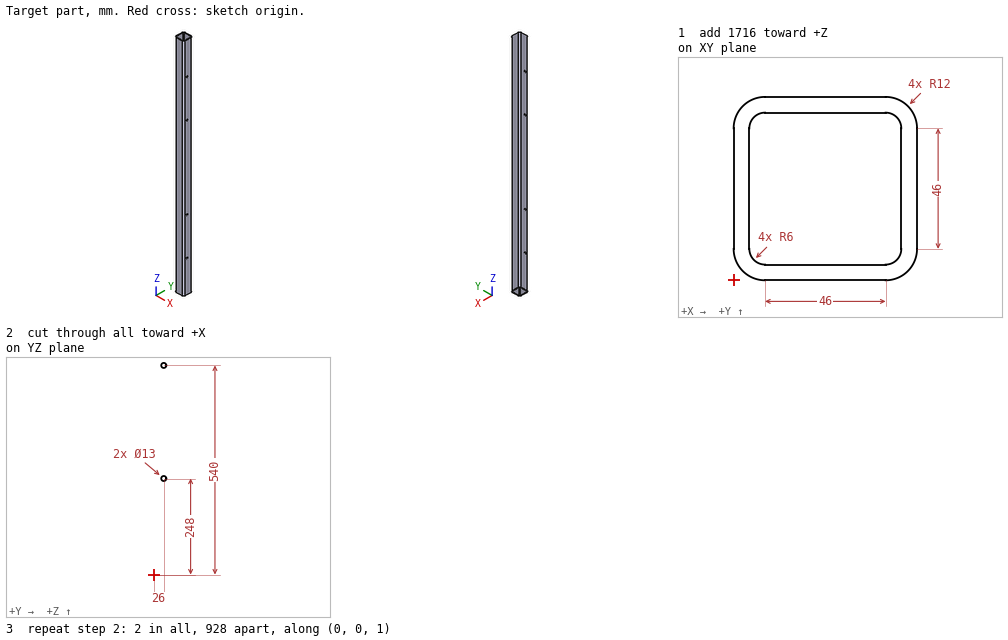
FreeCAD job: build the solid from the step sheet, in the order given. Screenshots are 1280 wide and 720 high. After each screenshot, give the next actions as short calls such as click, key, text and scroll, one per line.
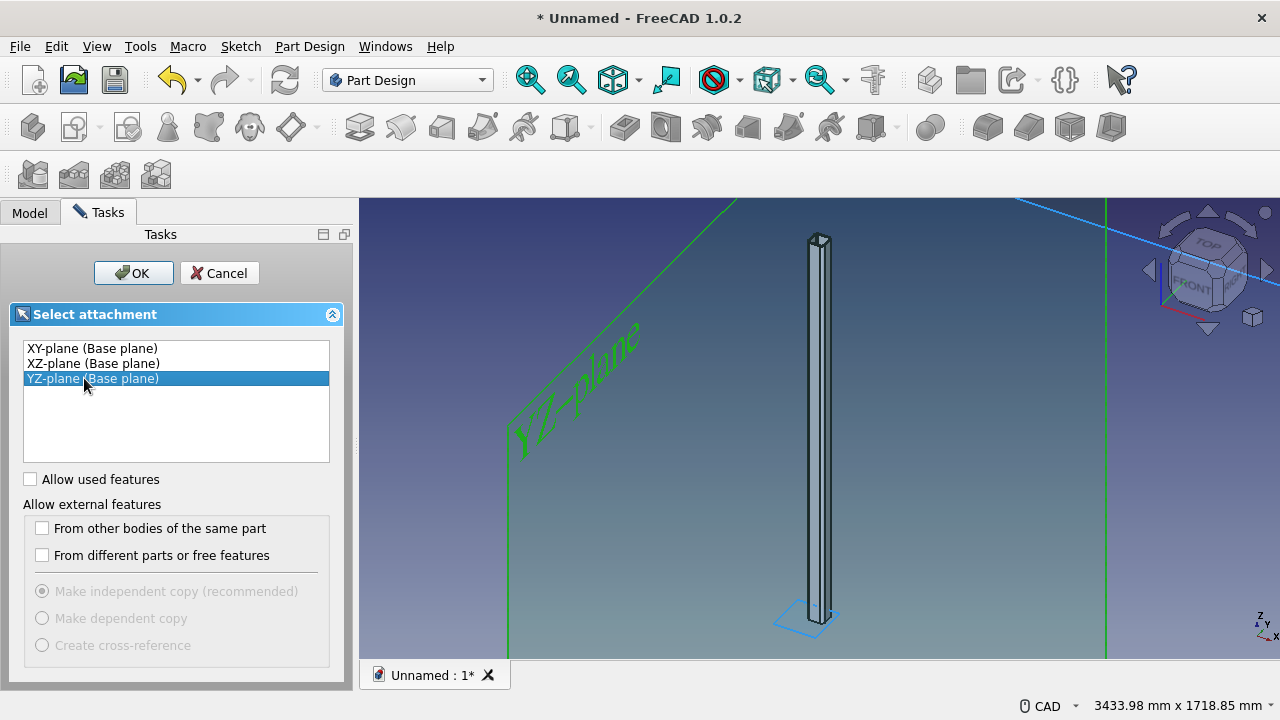
click(134, 273)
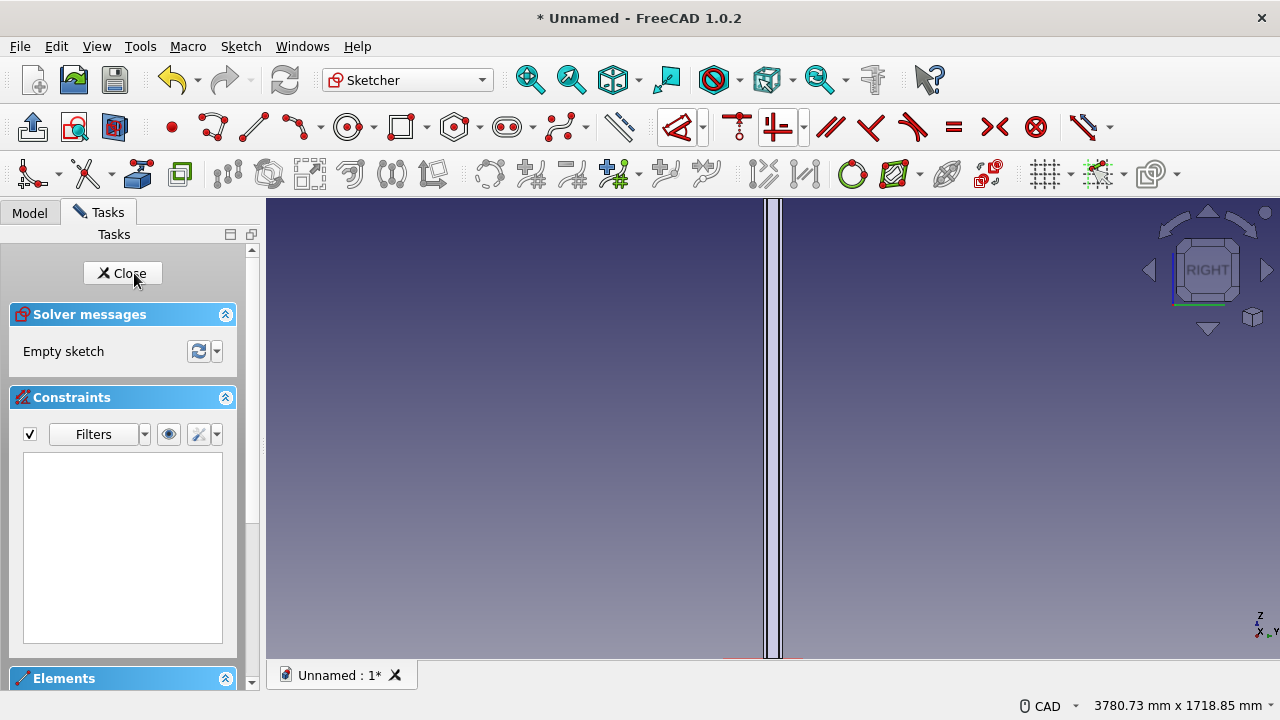
click(115, 128)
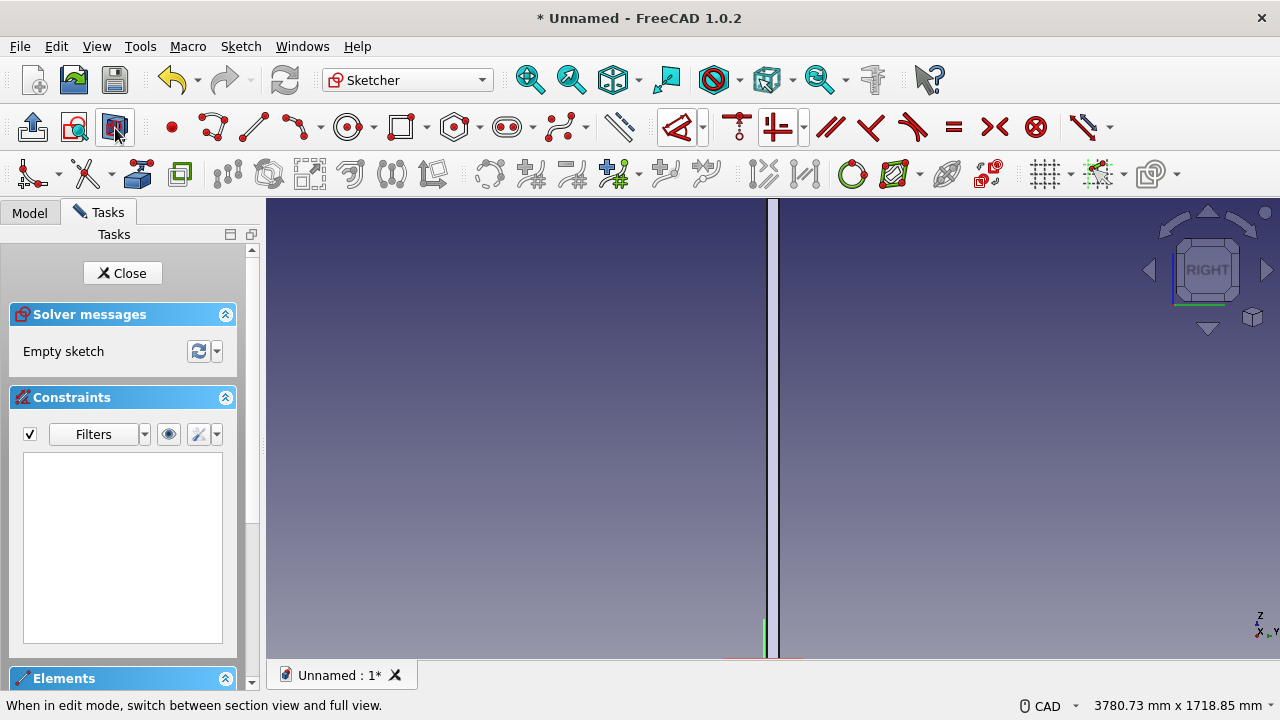
scroll(704, 428, down, 5)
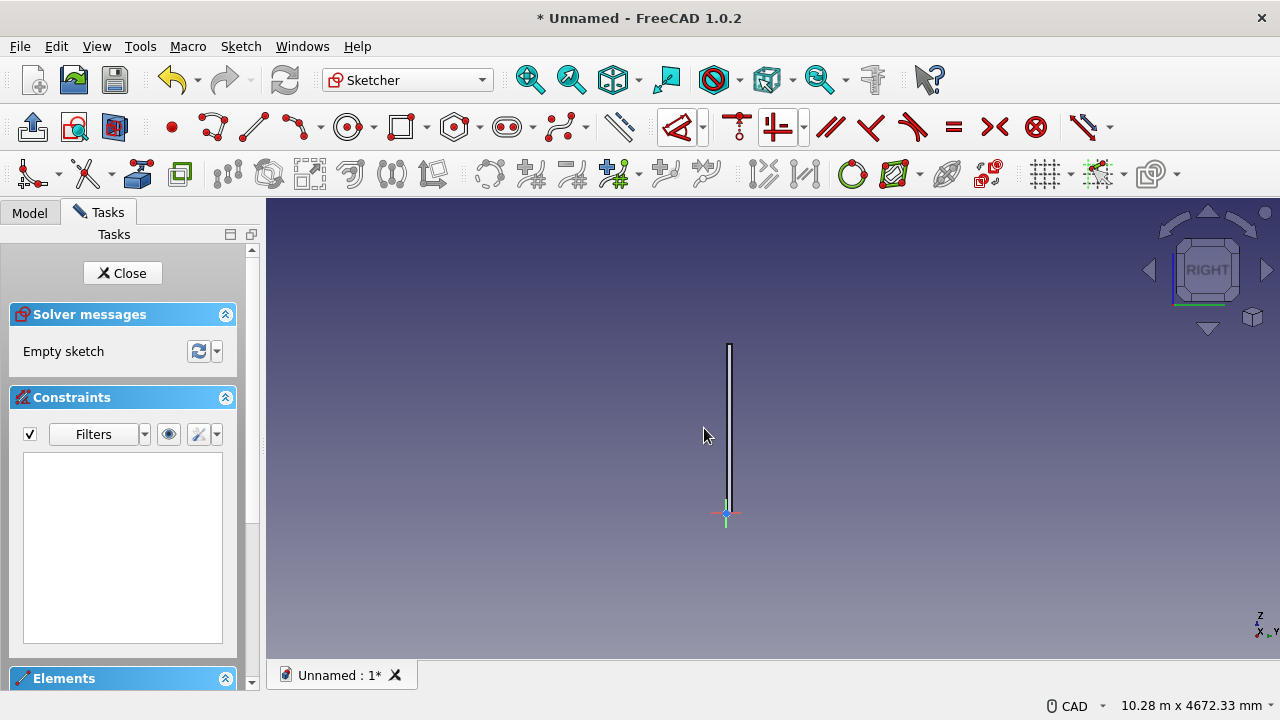
scroll(734, 501, up, 8)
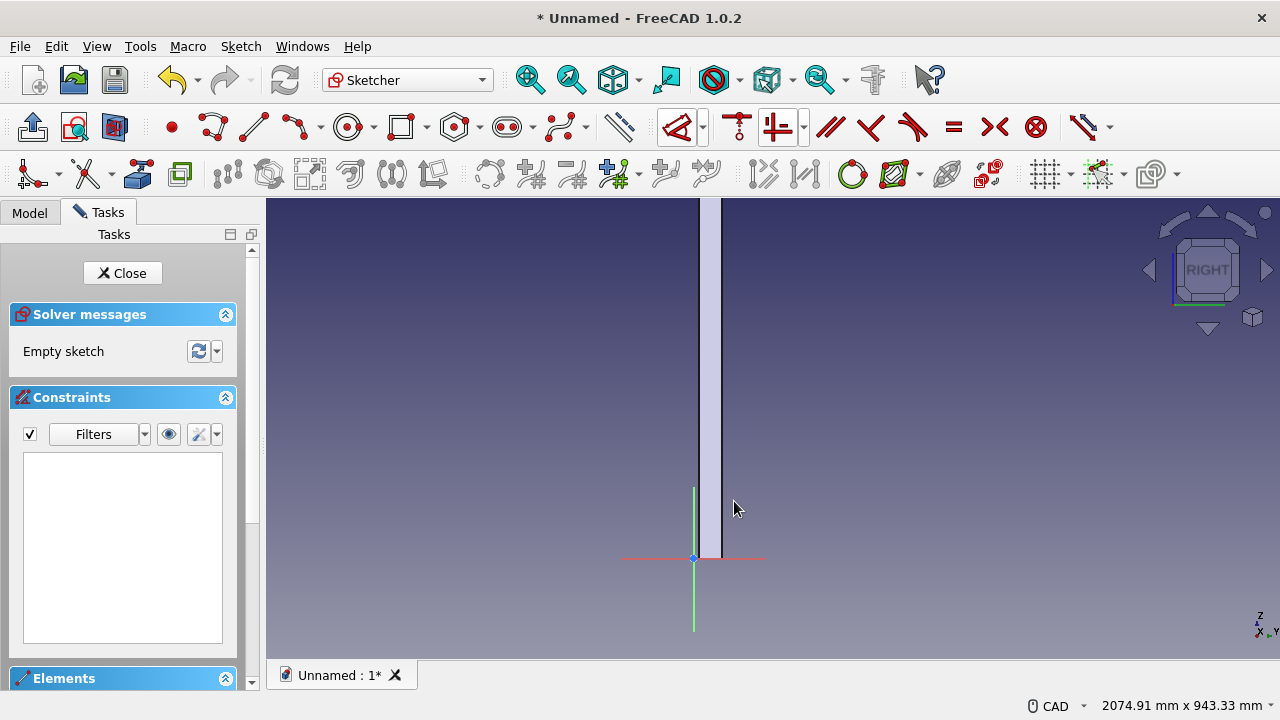
click(348, 128)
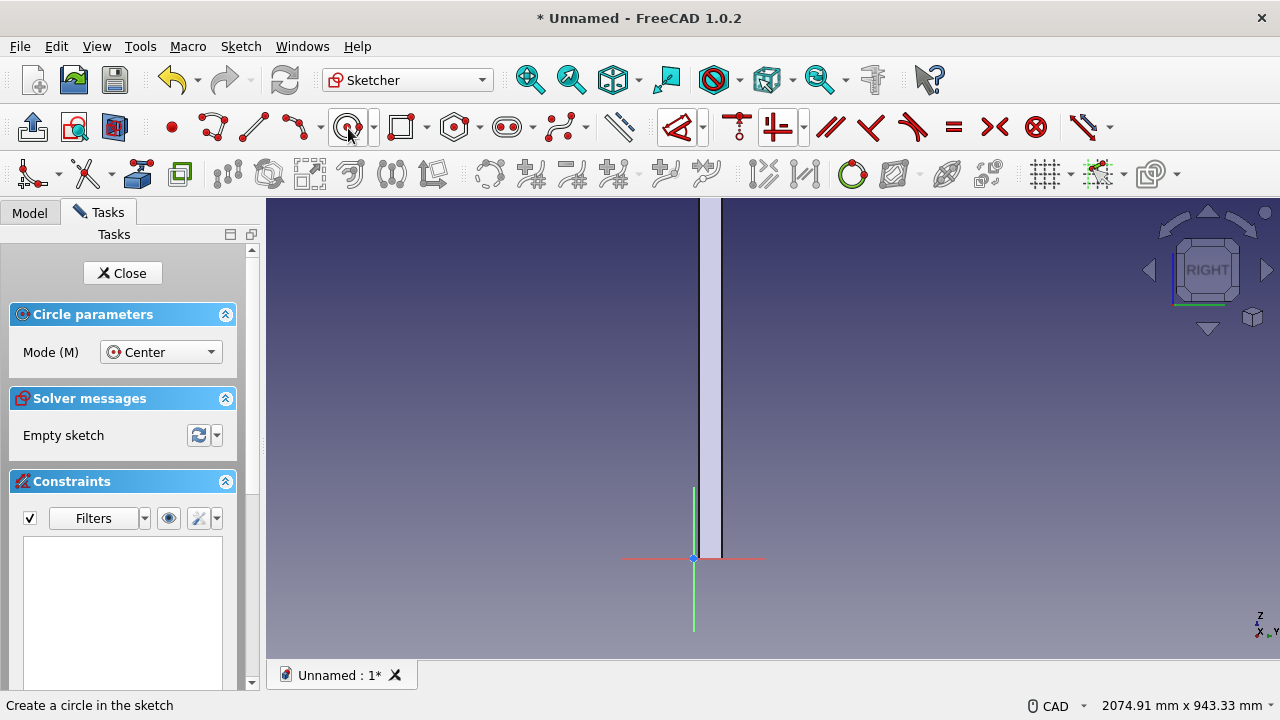
scroll(706, 437, up, 10)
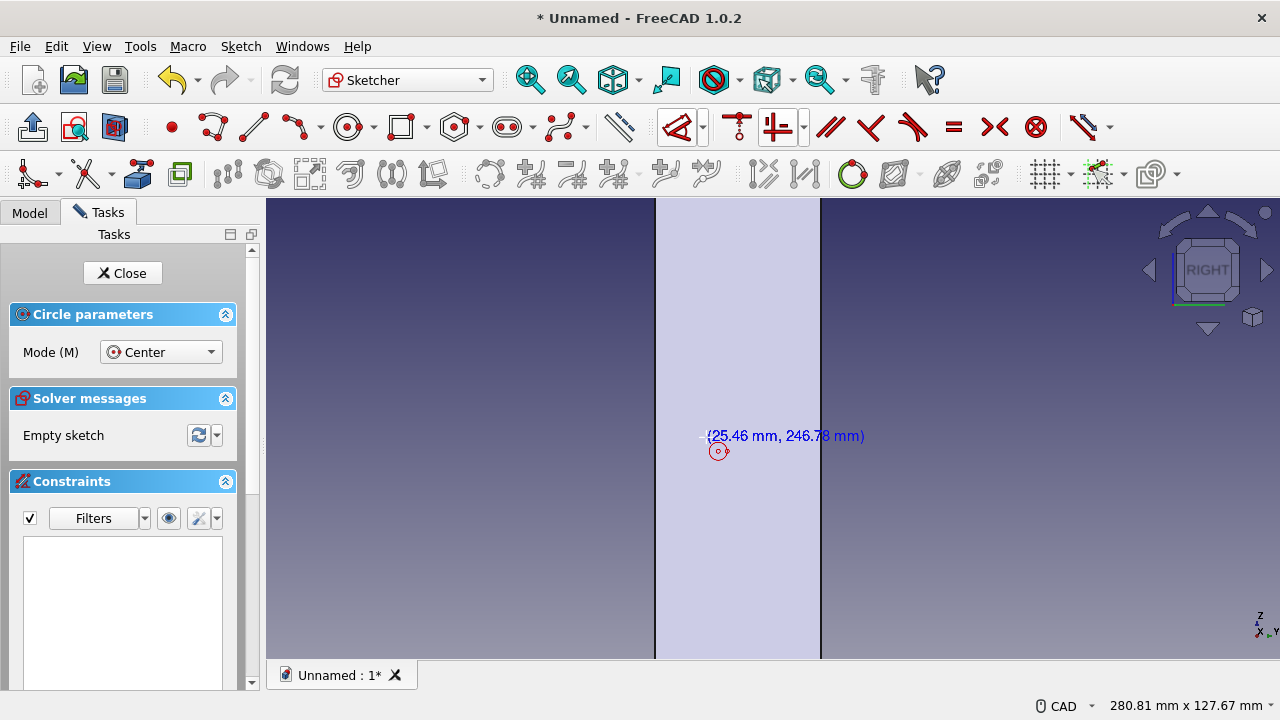
scroll(710, 441, down, 10)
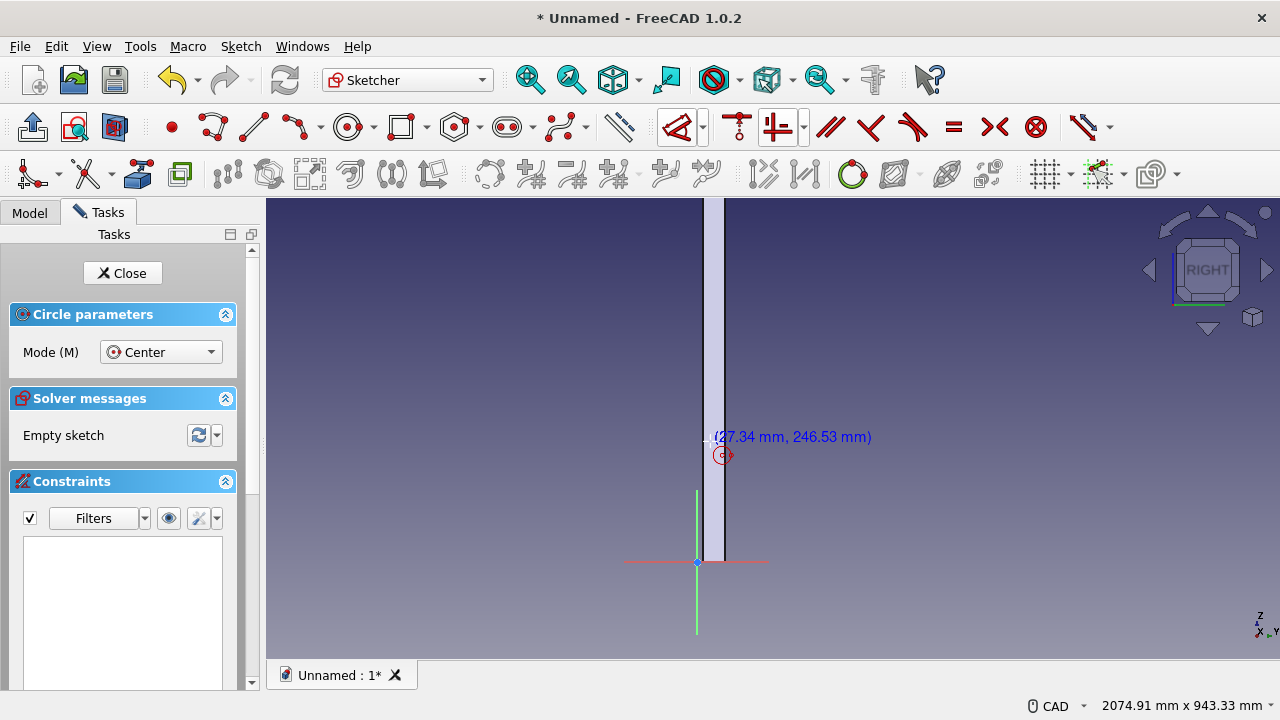
scroll(710, 441, up, 2)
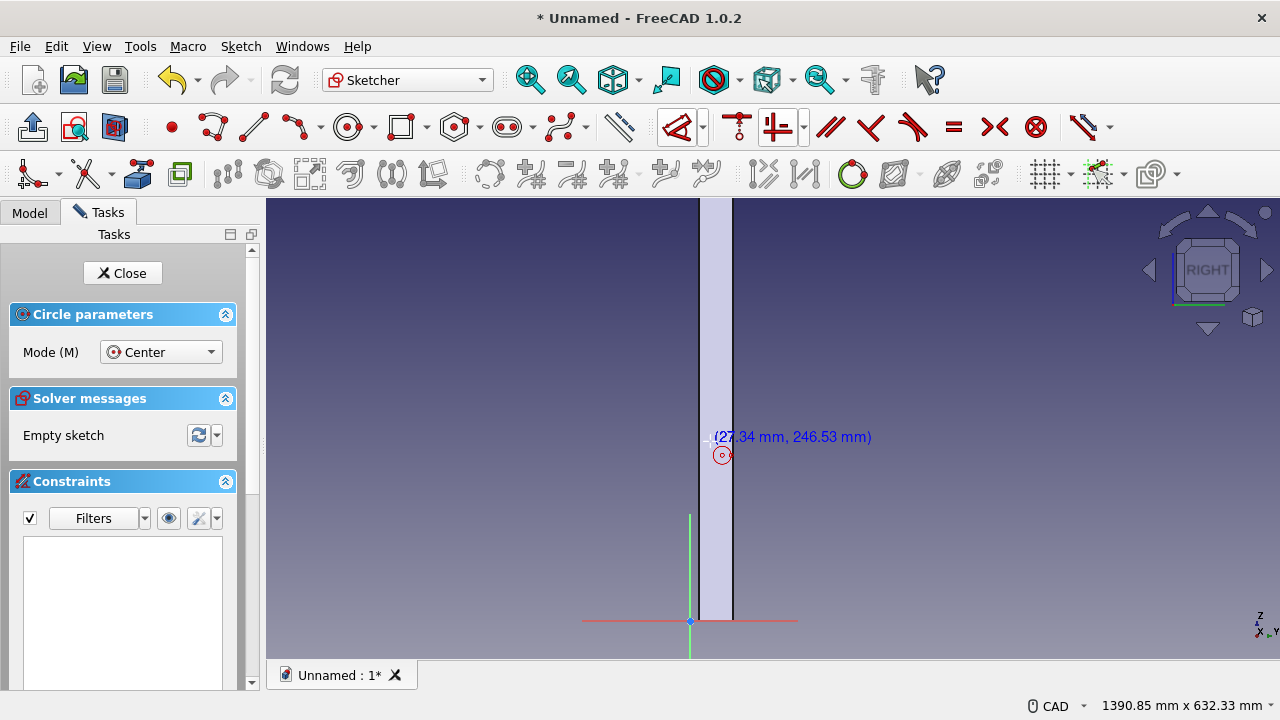
click(709, 441)
move(713, 437)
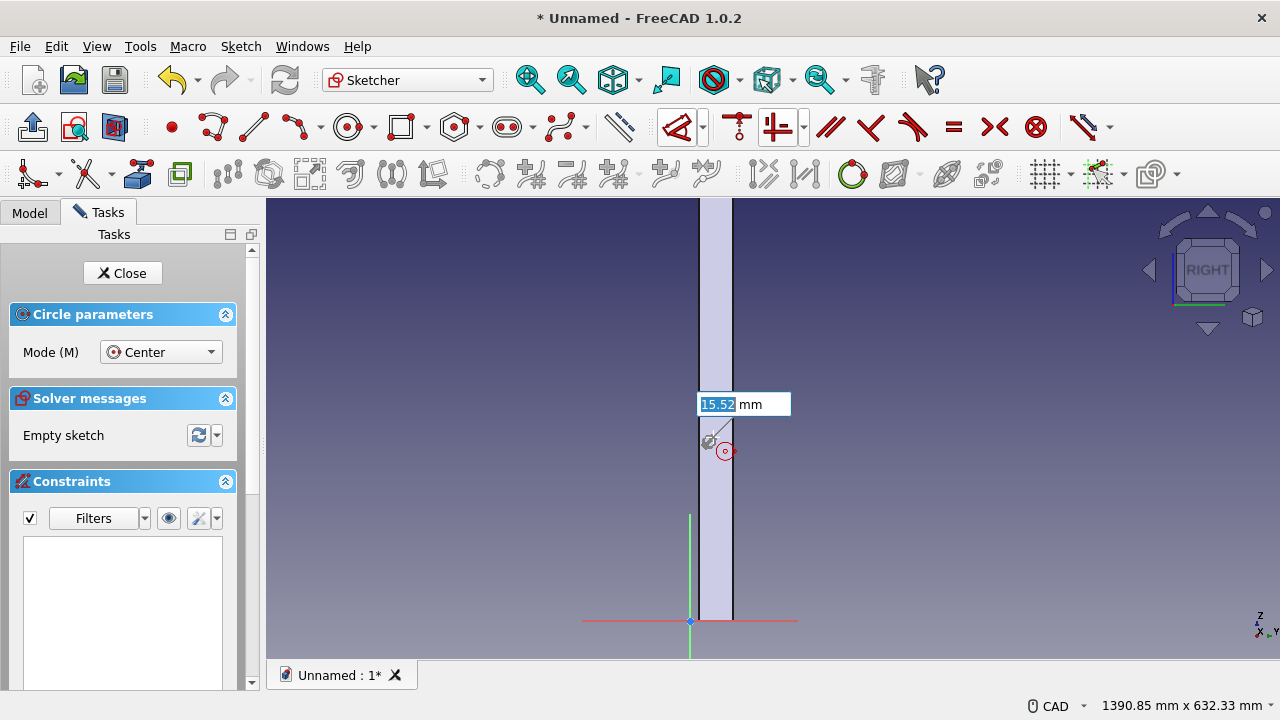
text(13)
key(Return)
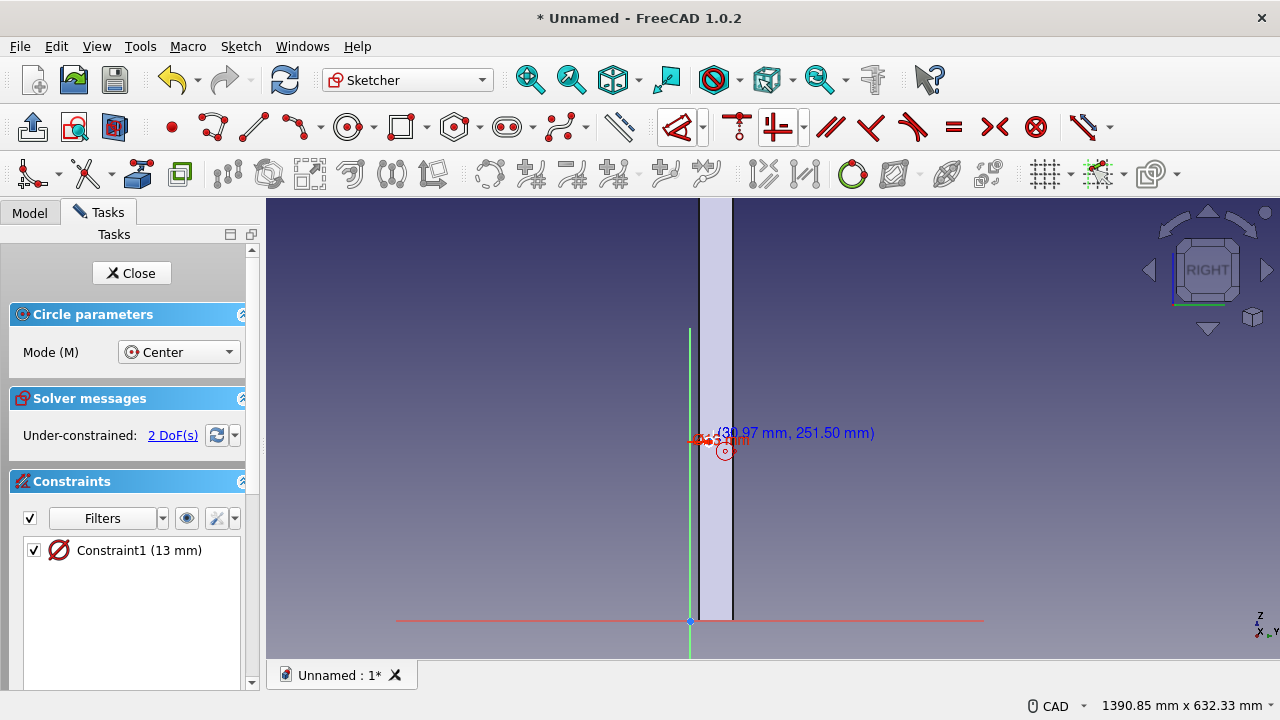
scroll(709, 228, up, 8)